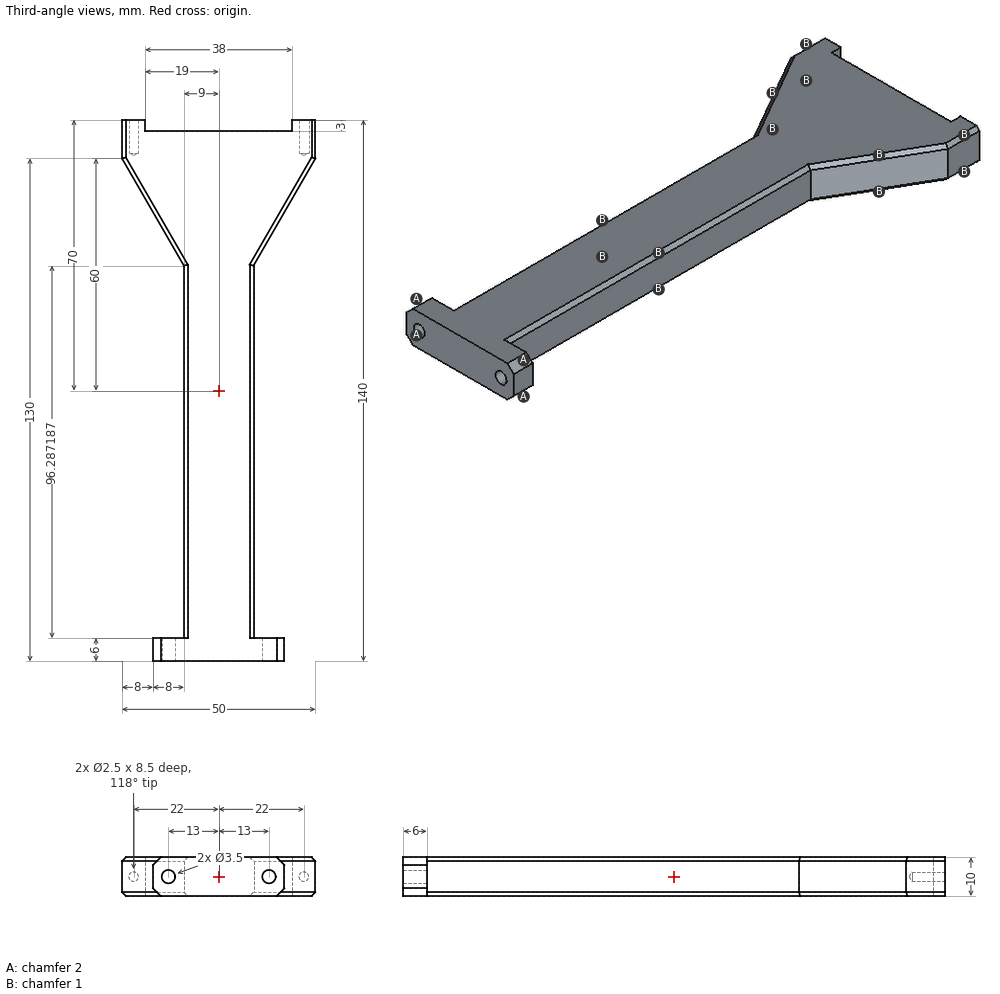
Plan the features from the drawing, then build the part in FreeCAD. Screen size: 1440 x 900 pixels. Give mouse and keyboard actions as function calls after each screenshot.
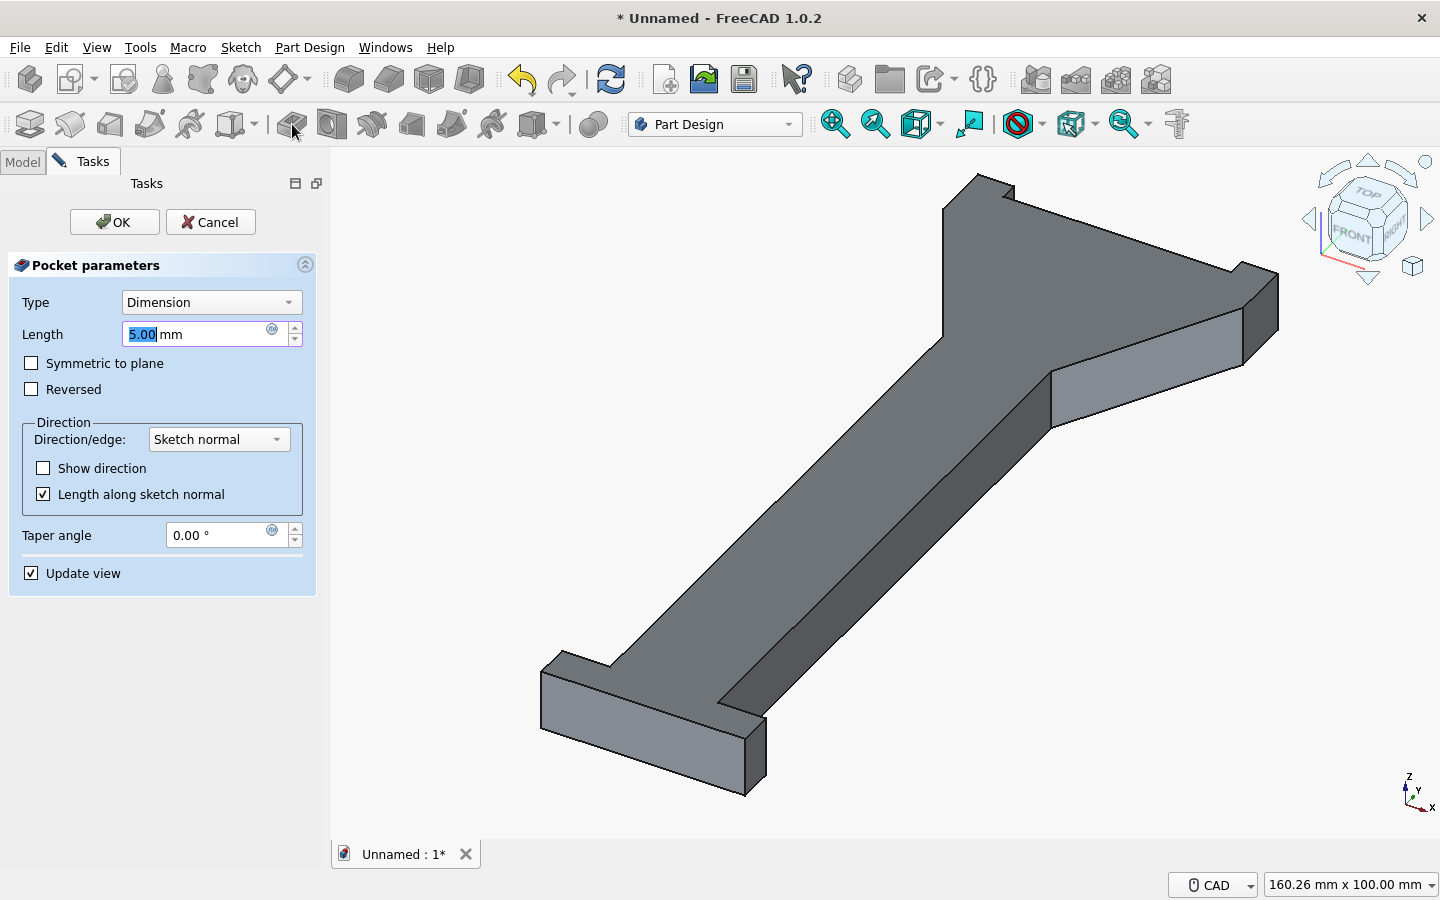
click(212, 302)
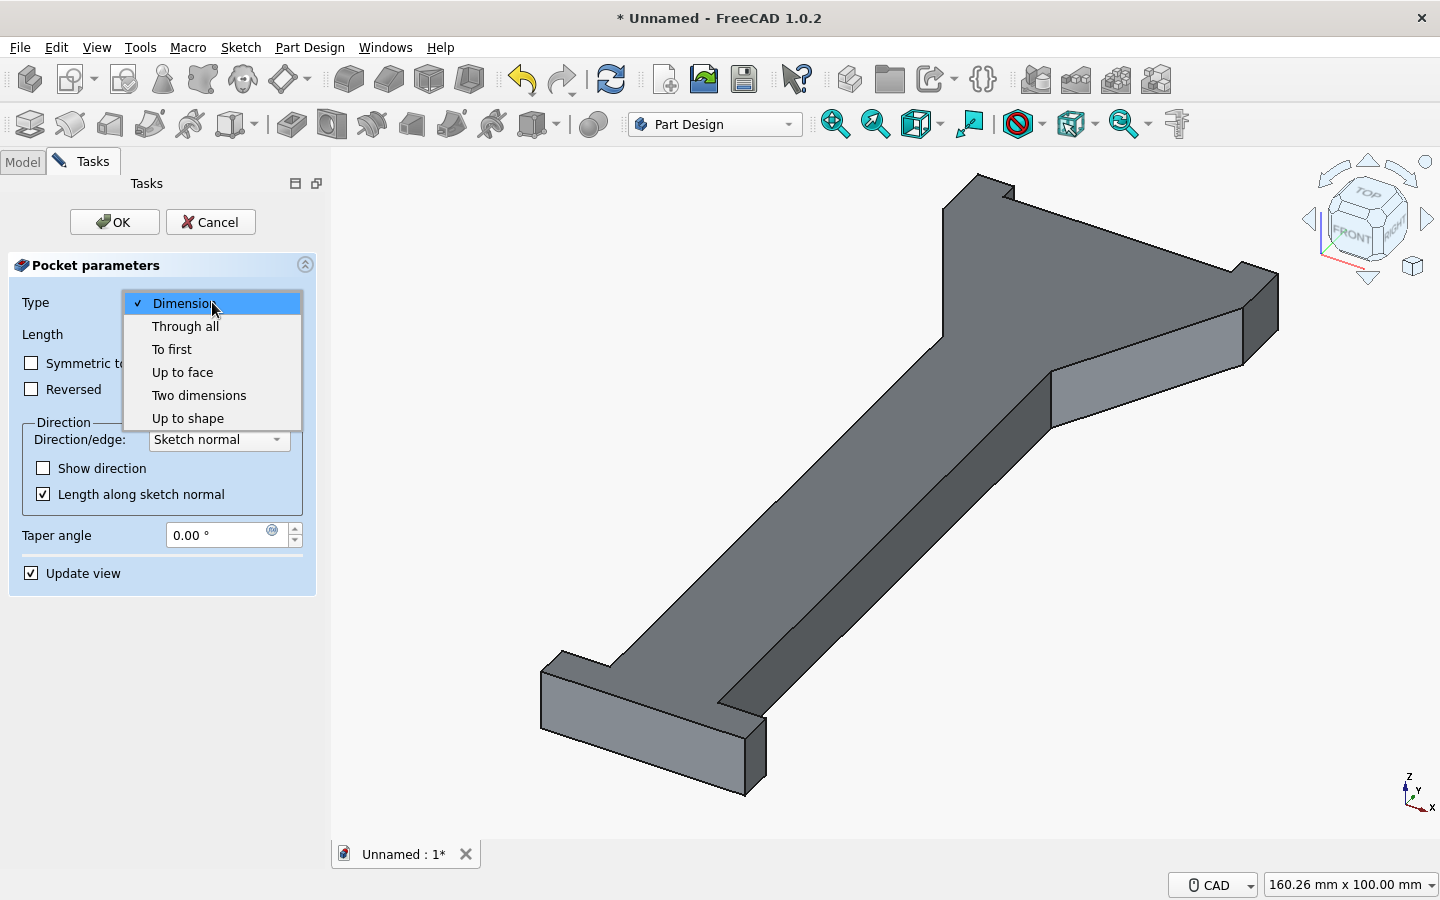
click(212, 326)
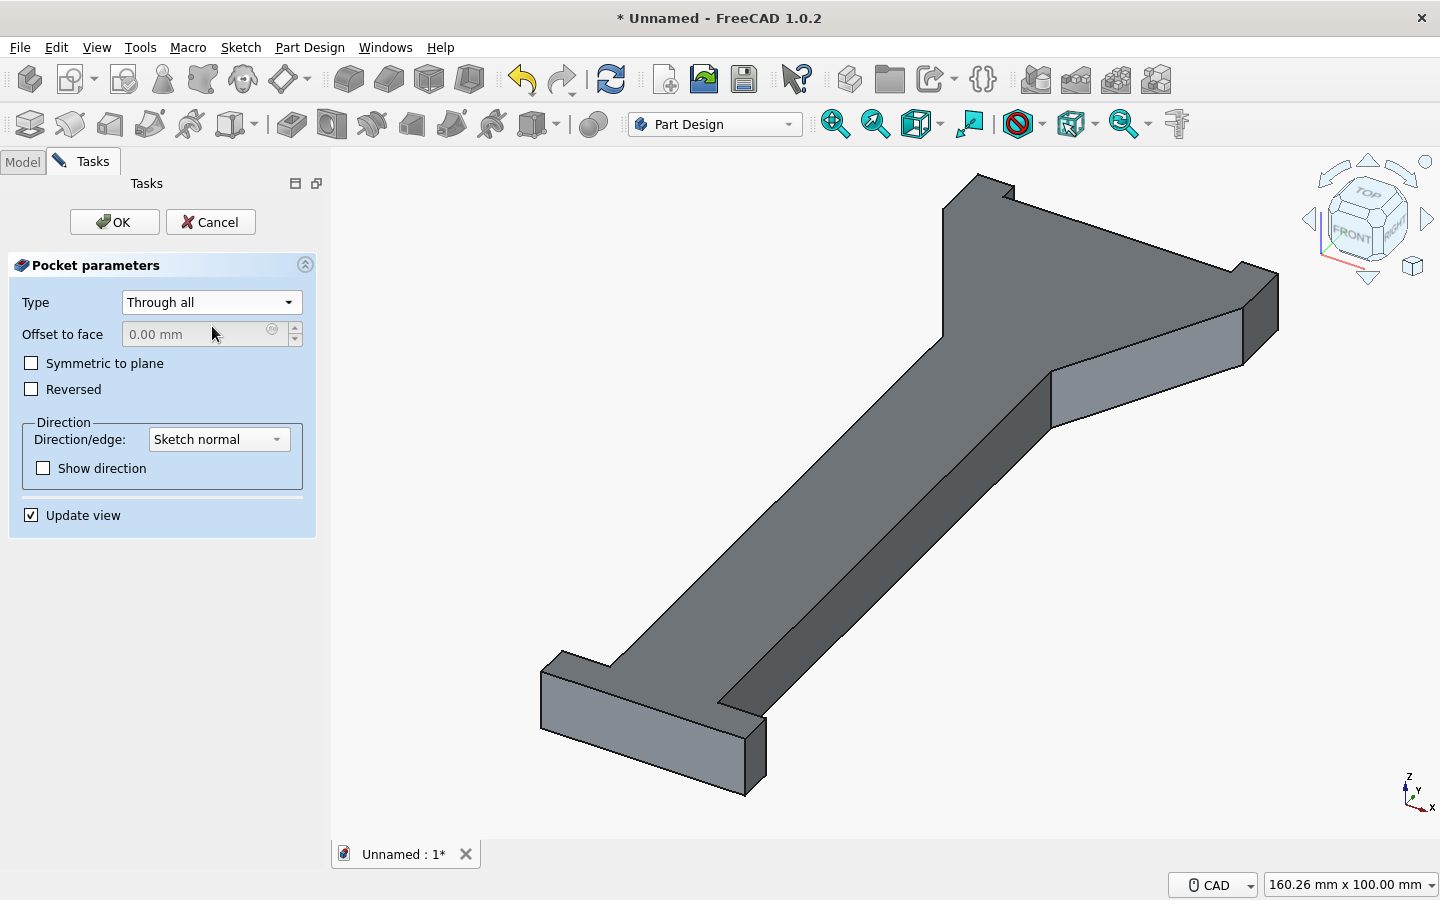
click(115, 222)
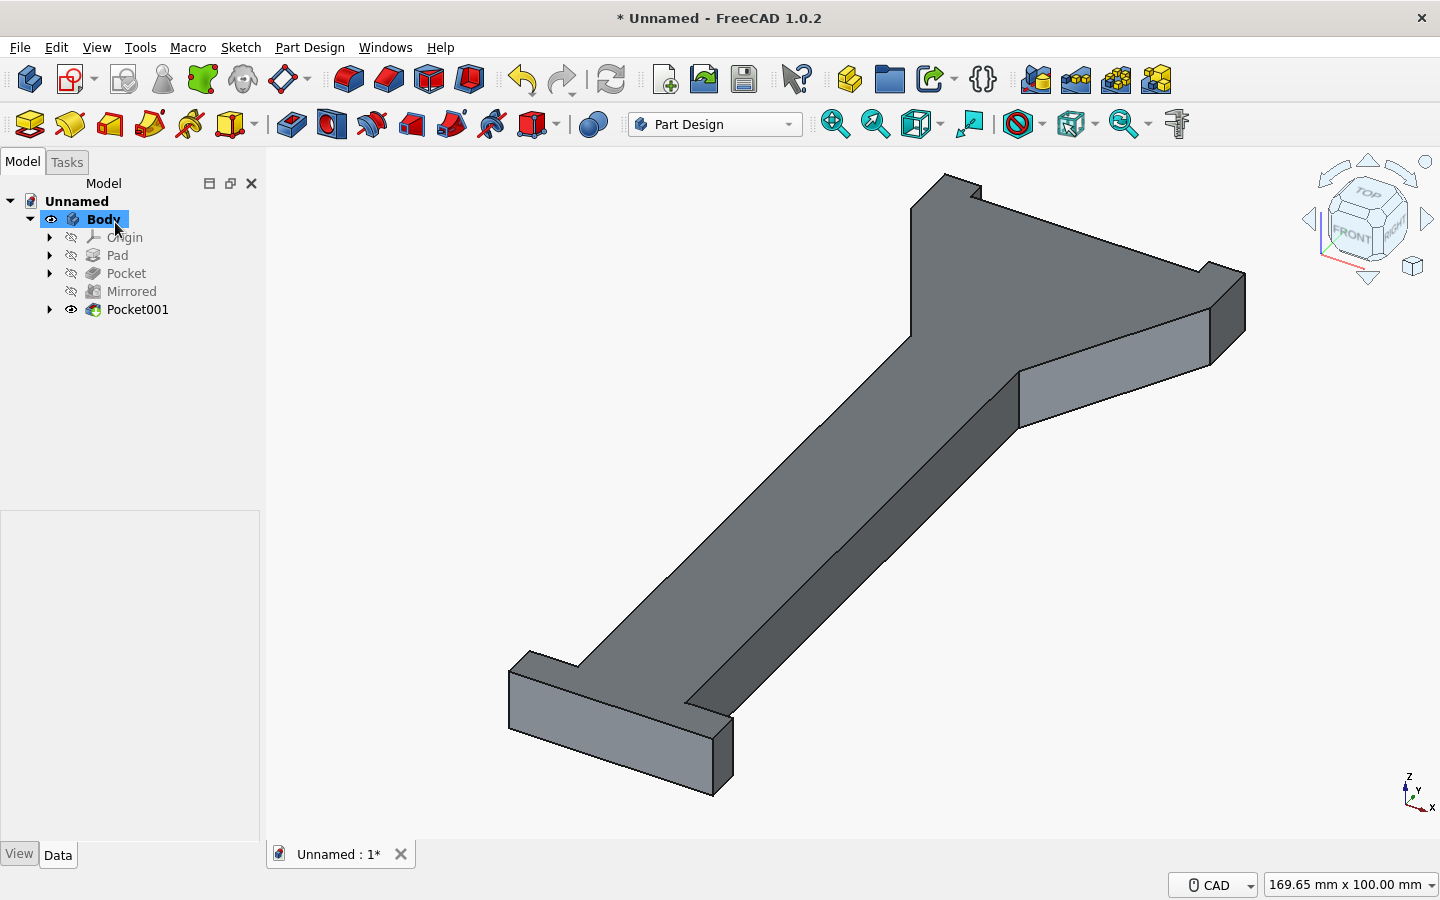
key(4)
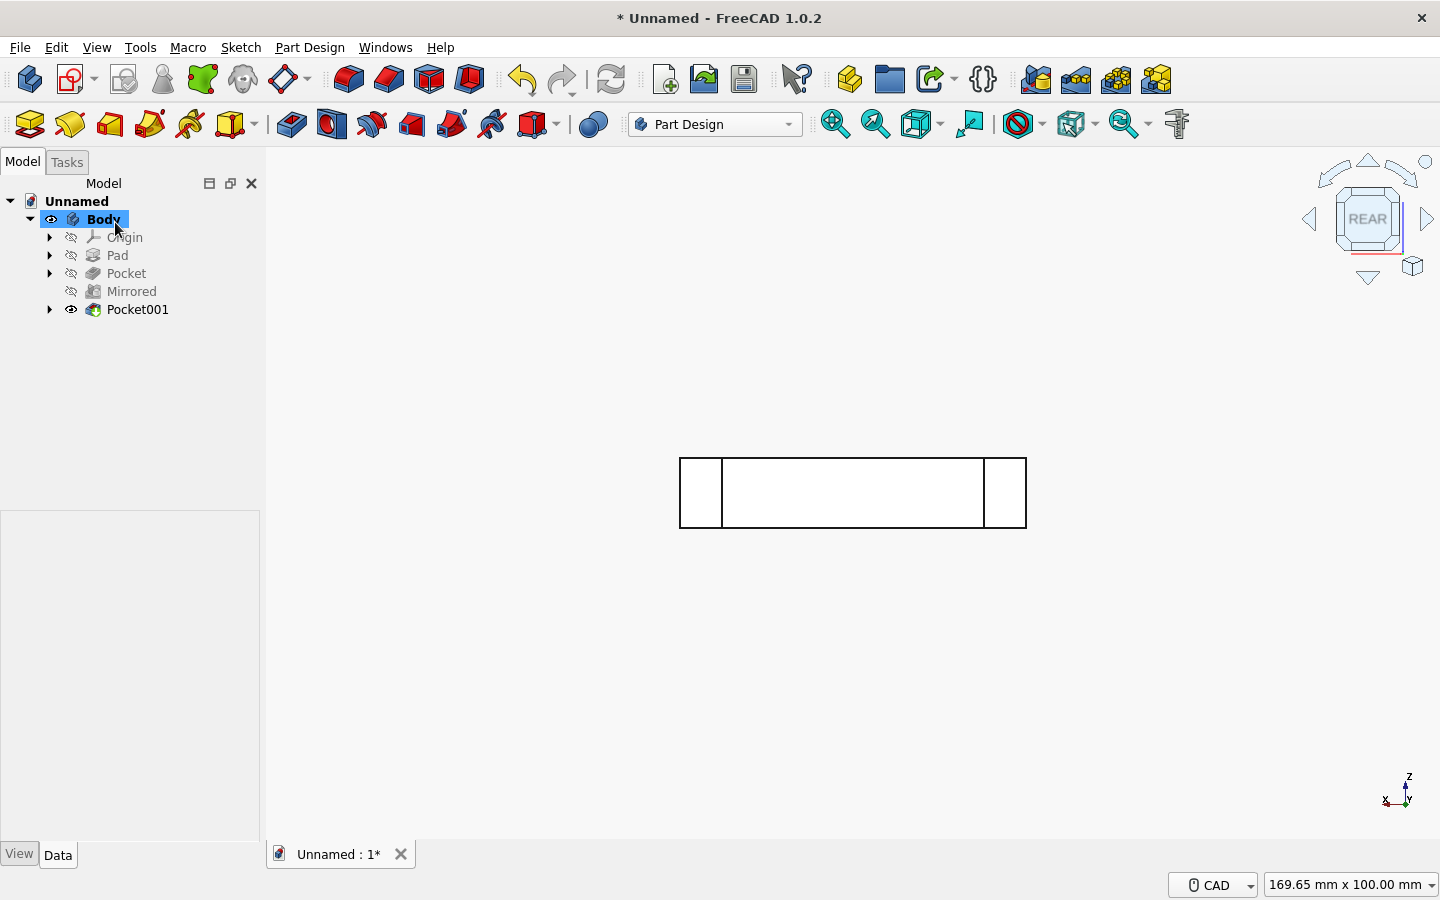
key(v)
key(f)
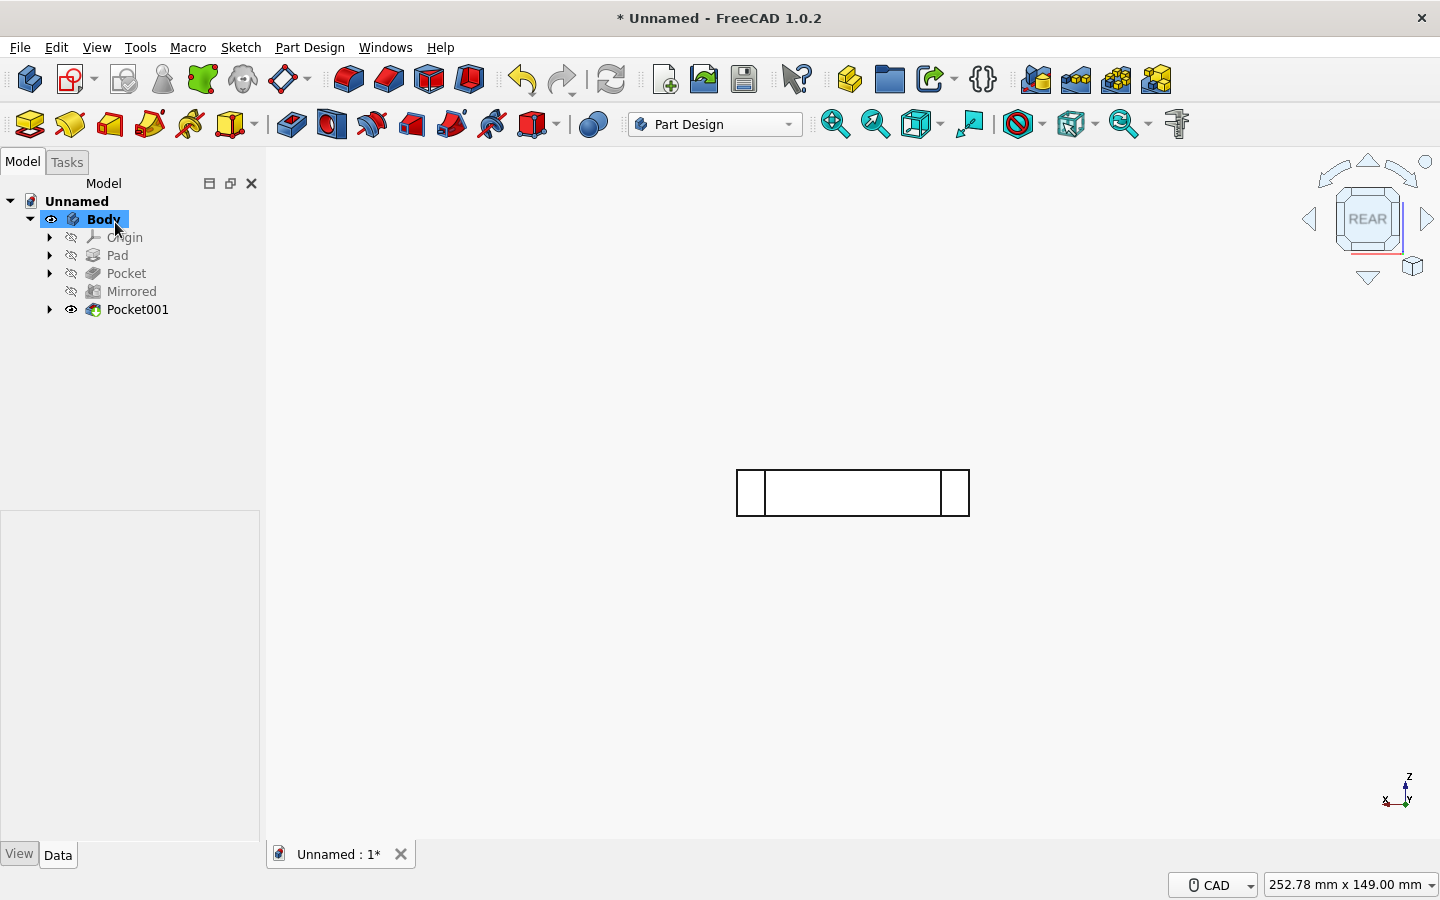
click(955, 485)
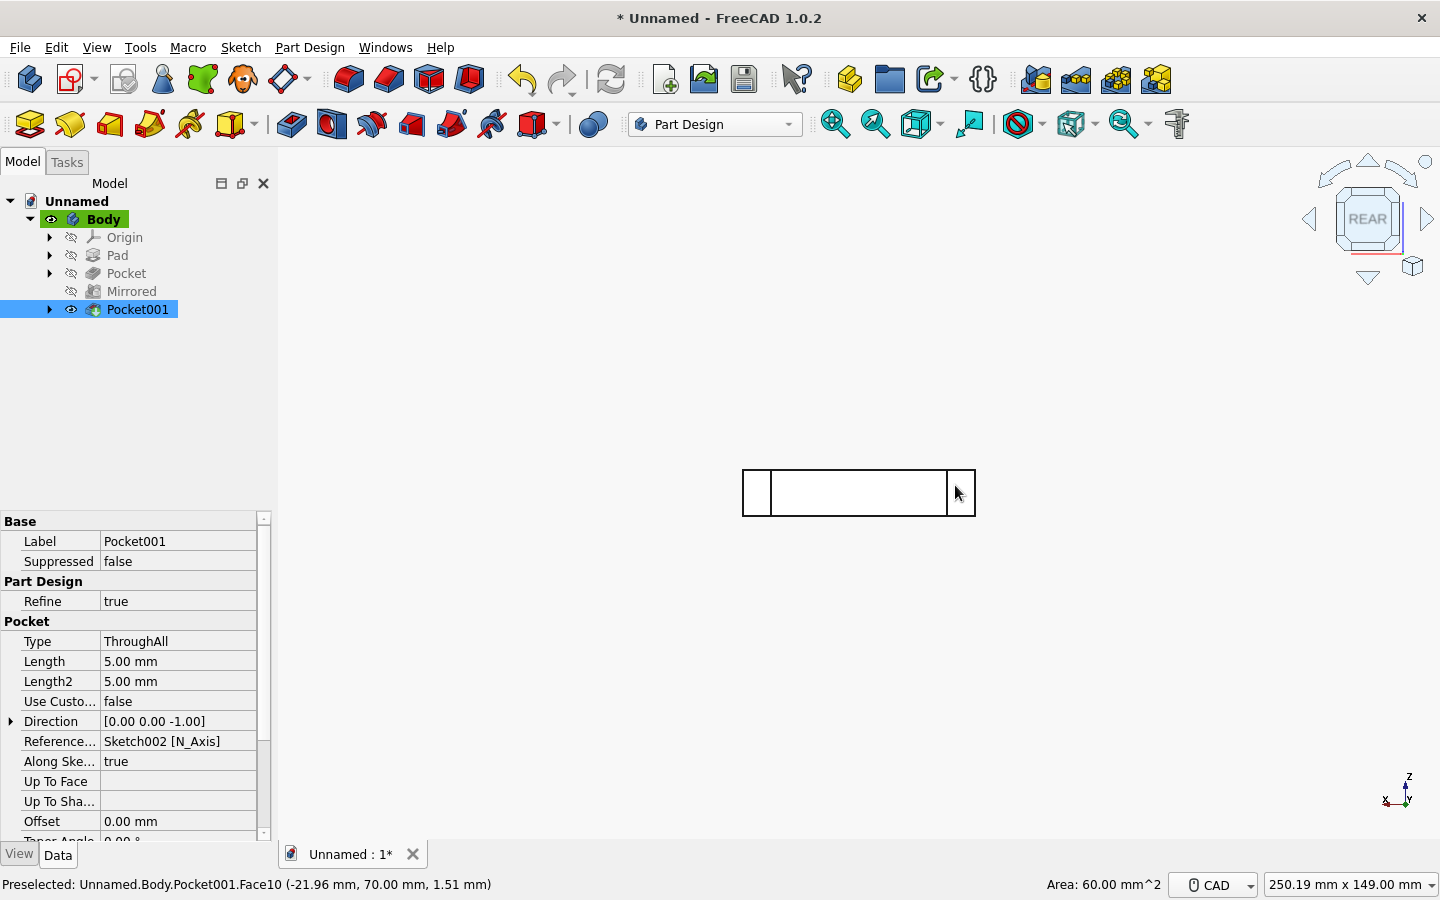
click(70, 80)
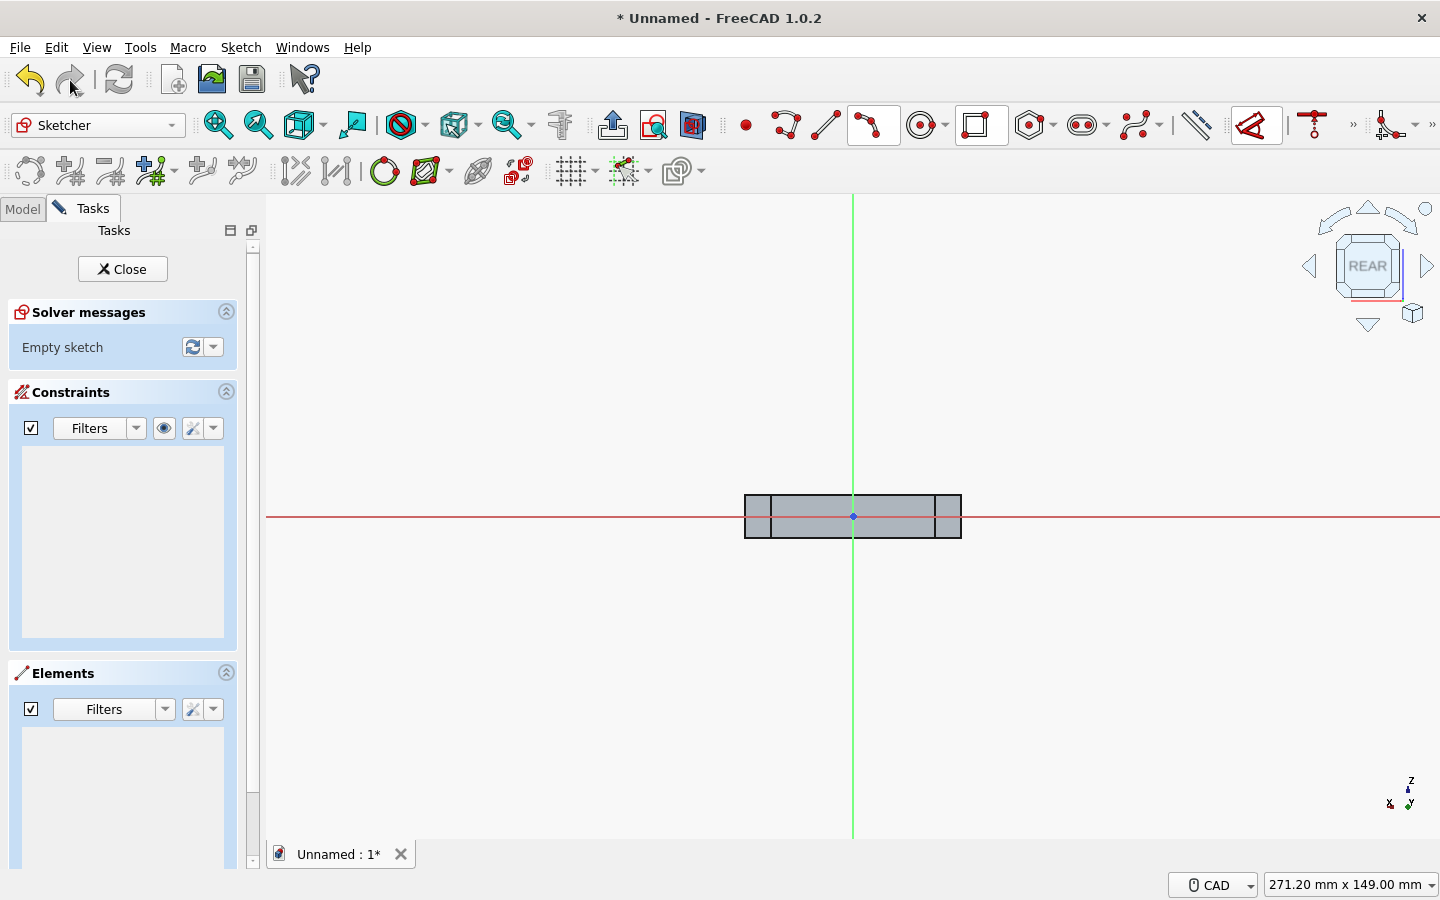
scroll(883, 516, up, 6)